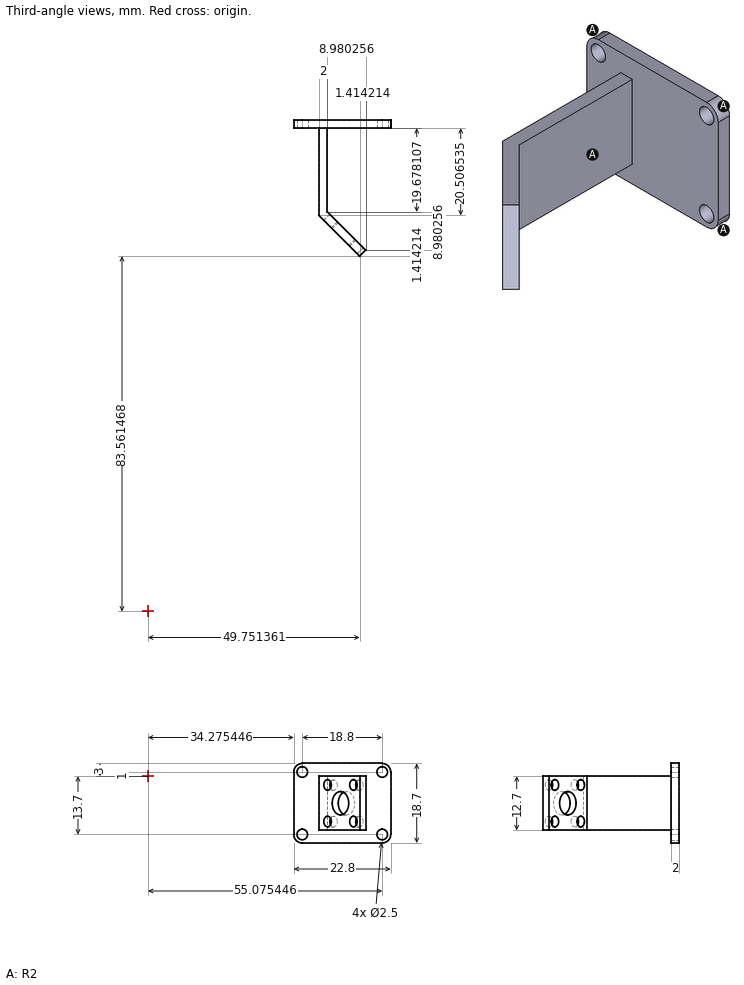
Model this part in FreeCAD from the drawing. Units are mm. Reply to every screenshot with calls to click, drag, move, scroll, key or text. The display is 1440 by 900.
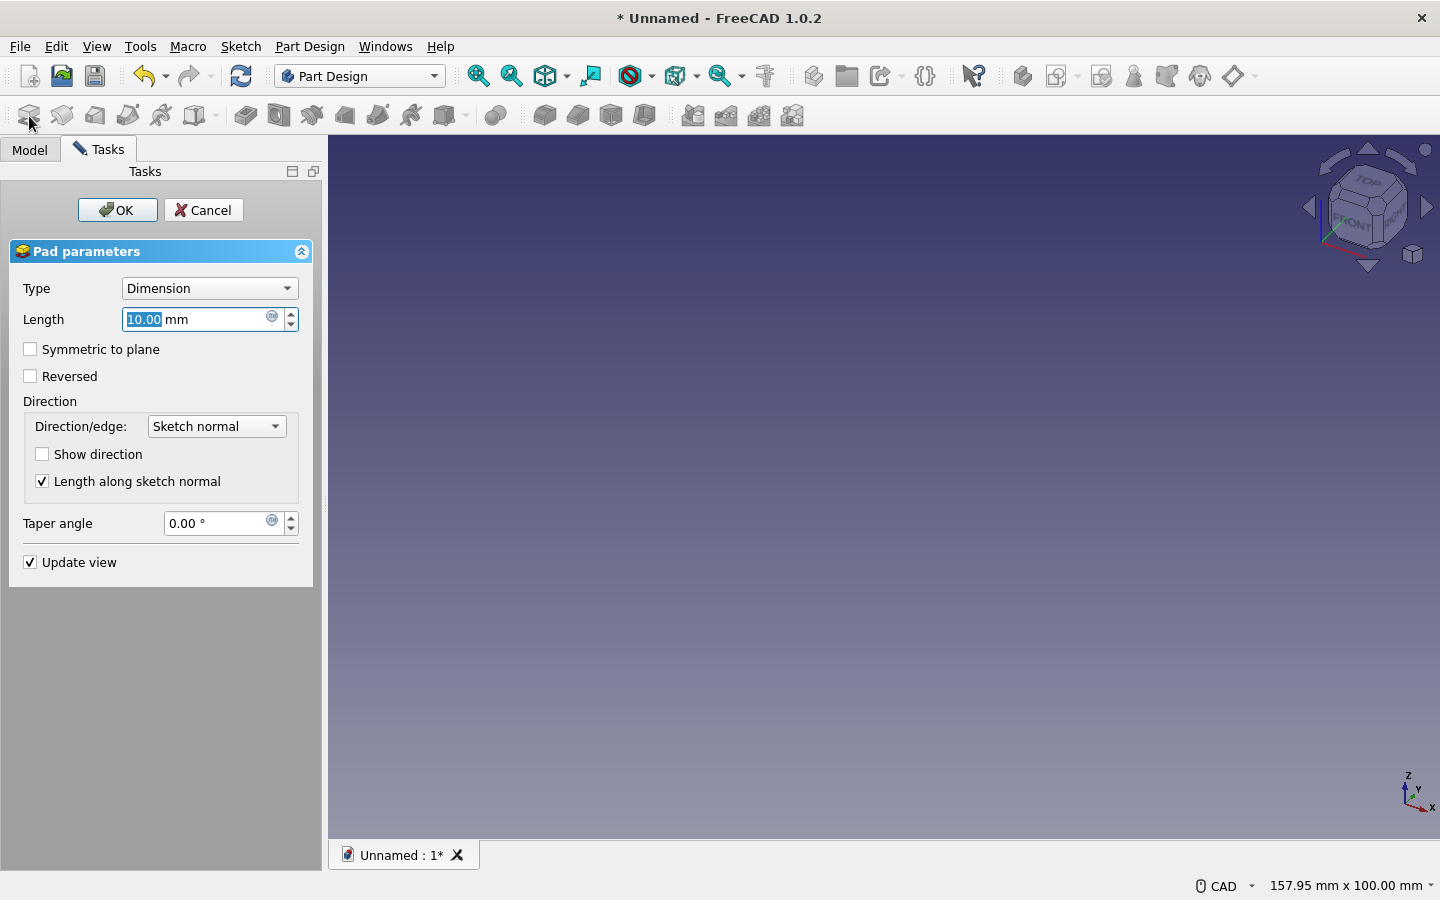
text(12.7)
key(Tab)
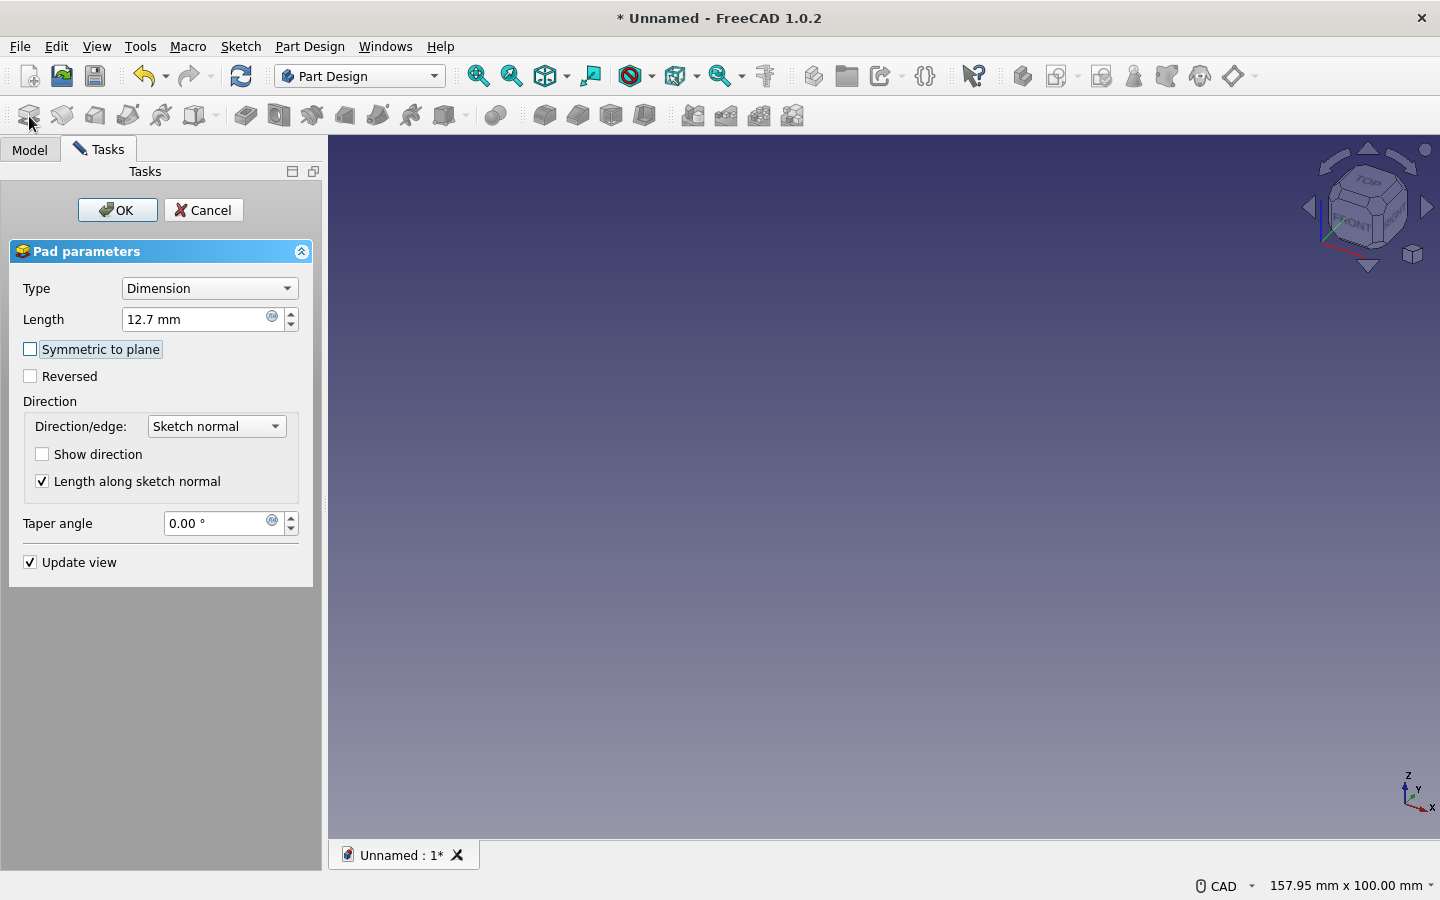
click(31, 376)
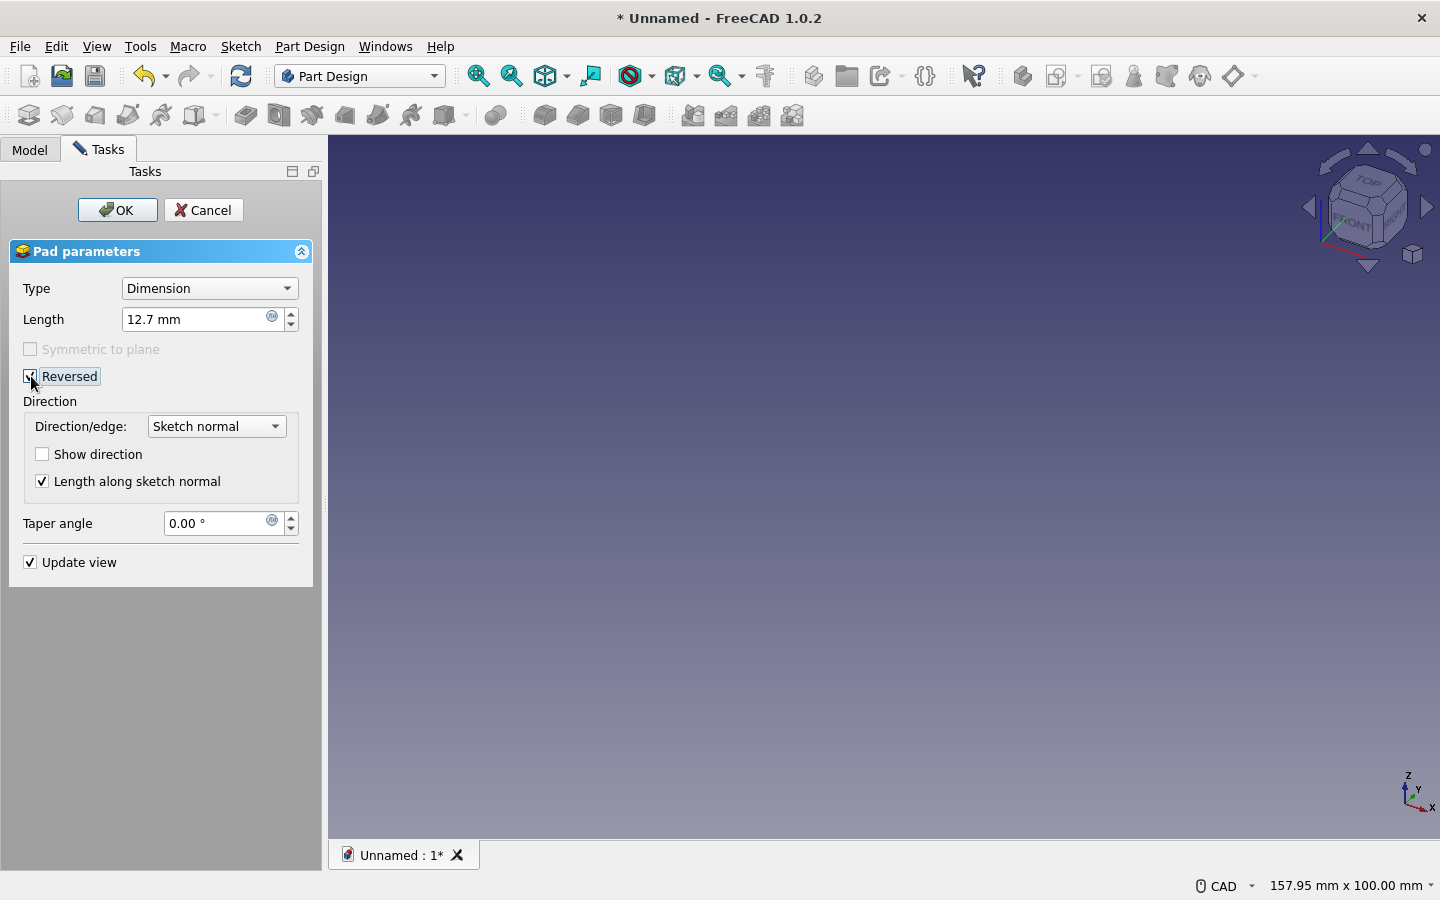
click(118, 210)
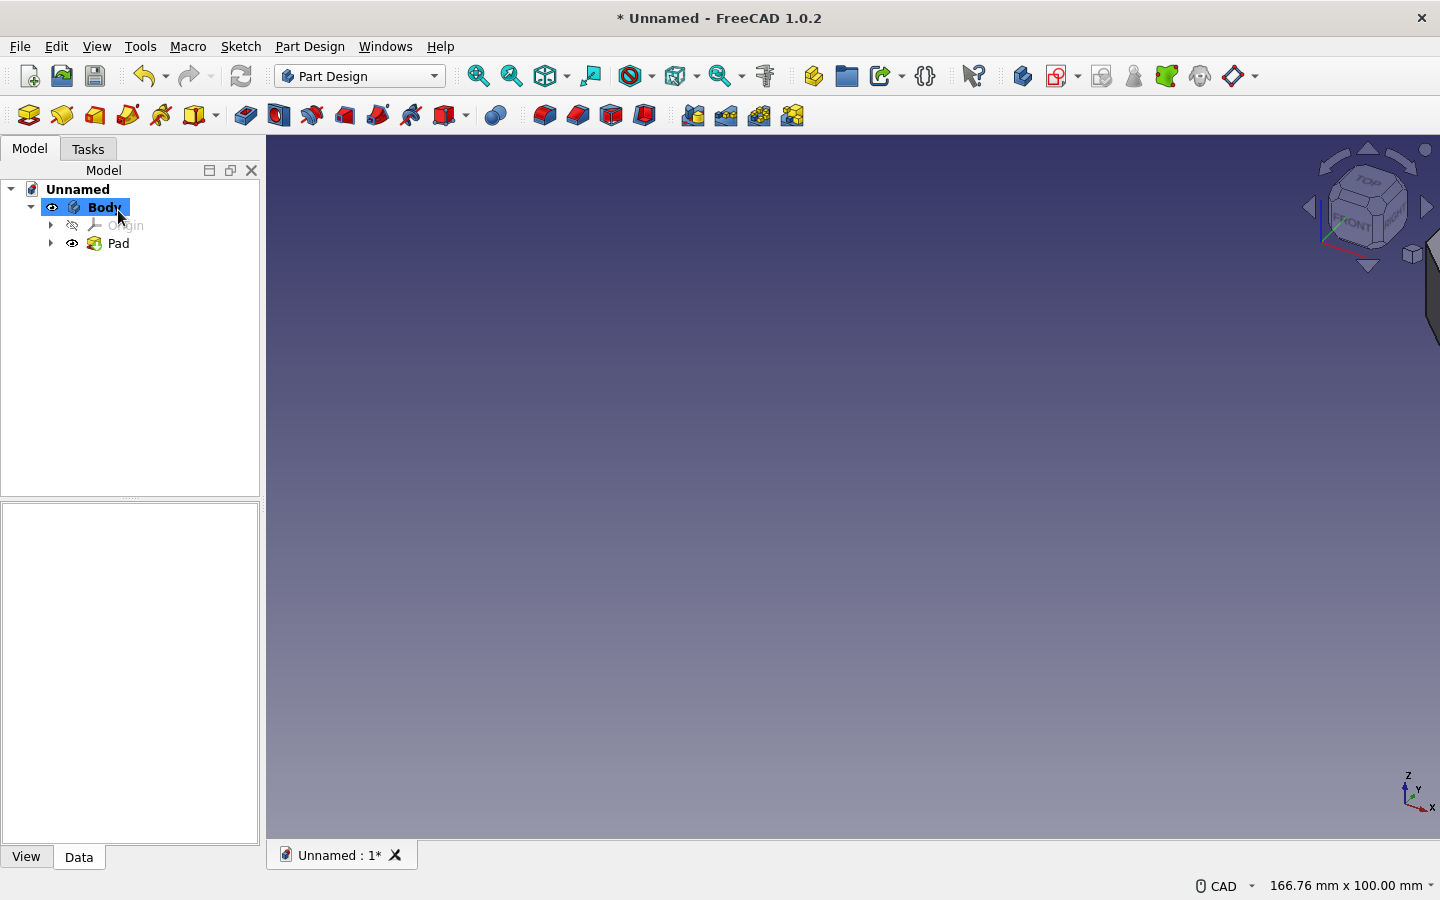
click(479, 76)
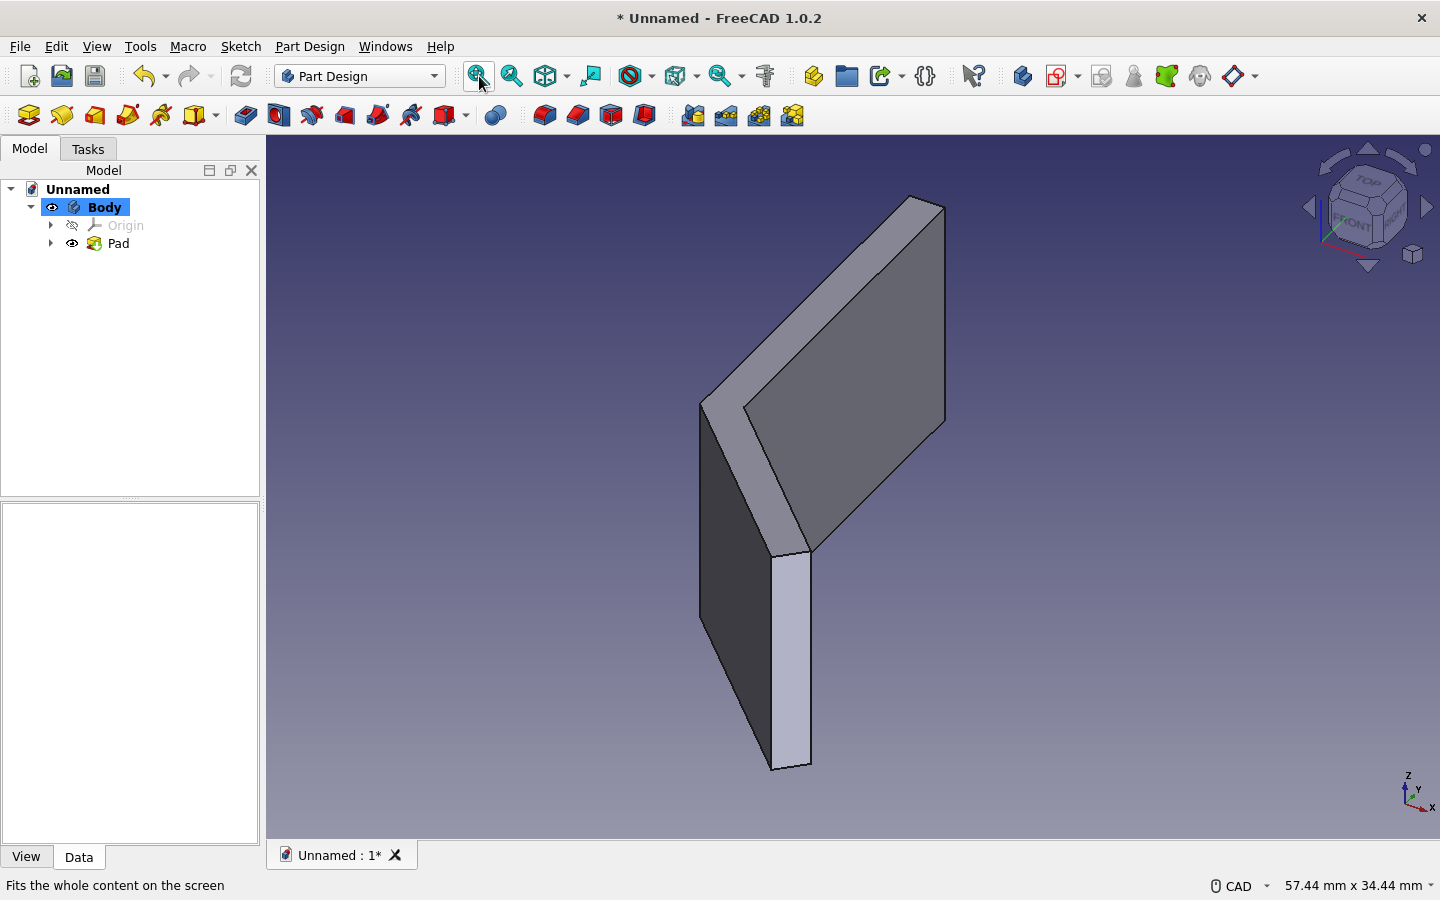
key(4)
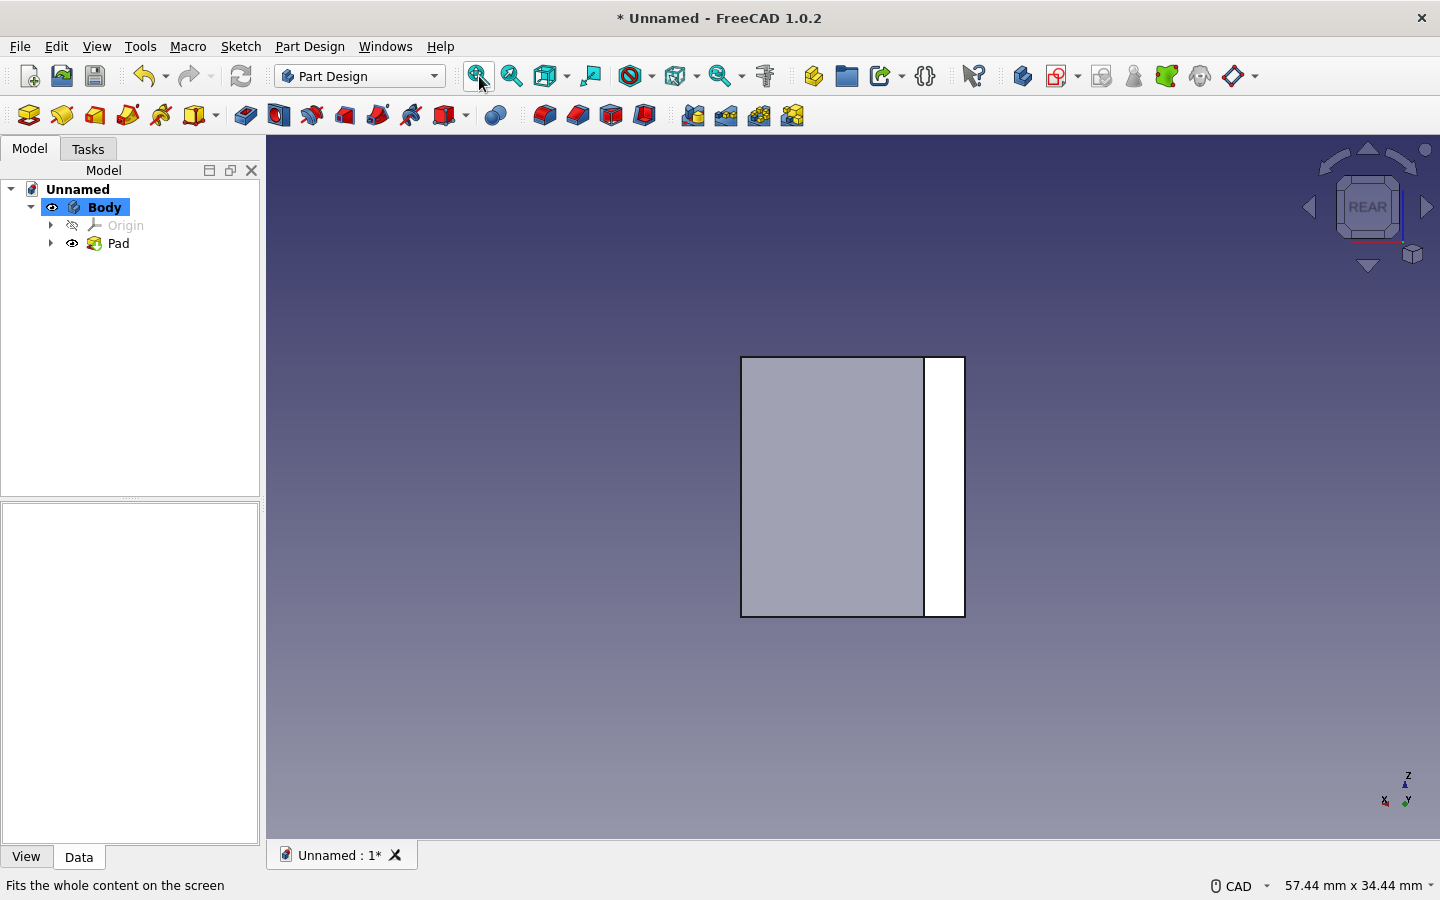
click(479, 76)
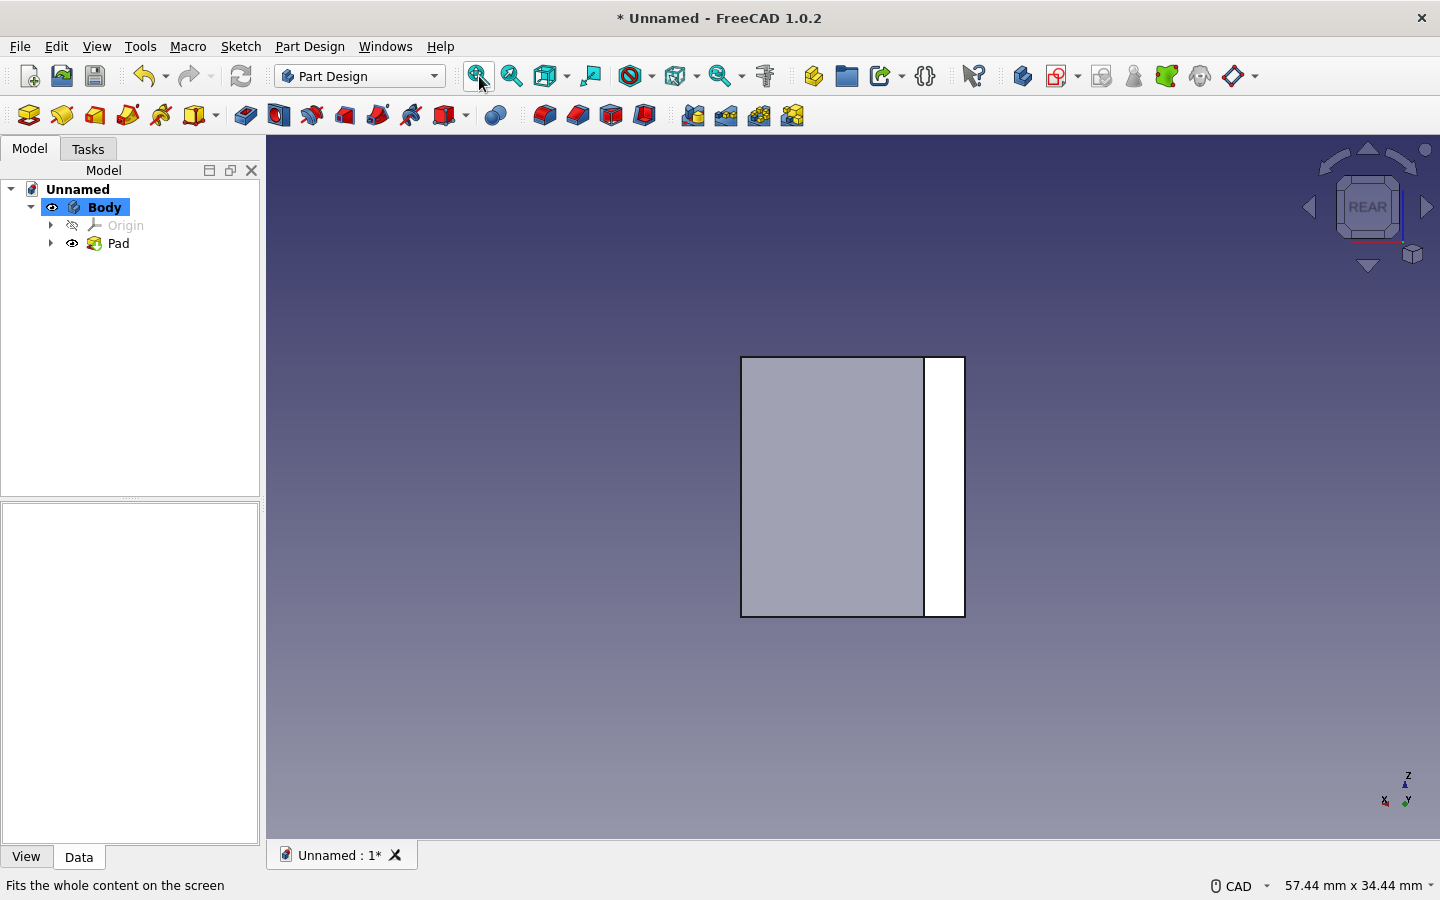
click(833, 486)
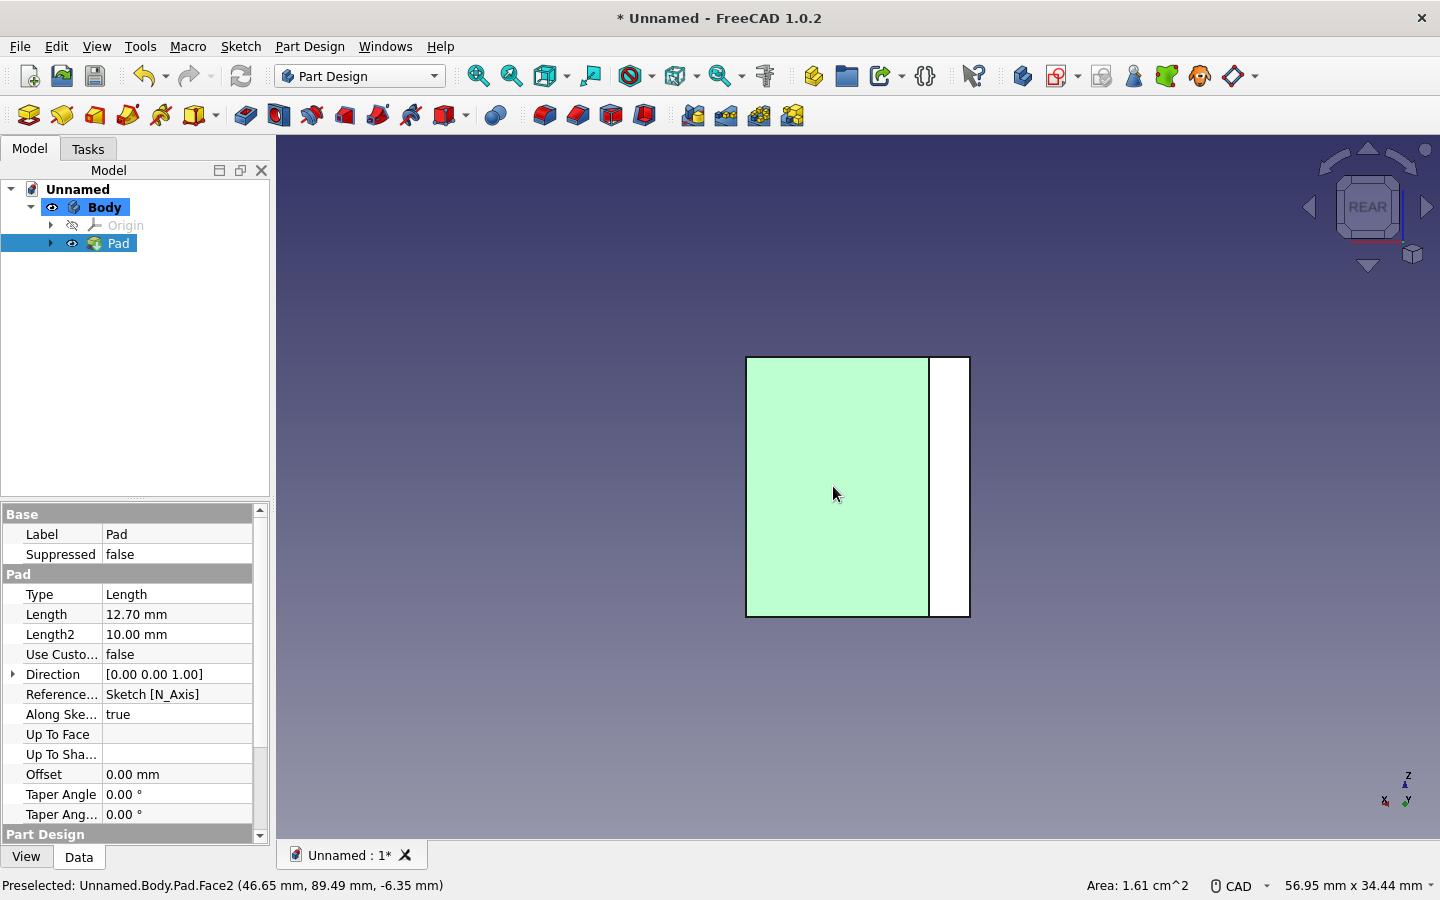
click(1056, 76)